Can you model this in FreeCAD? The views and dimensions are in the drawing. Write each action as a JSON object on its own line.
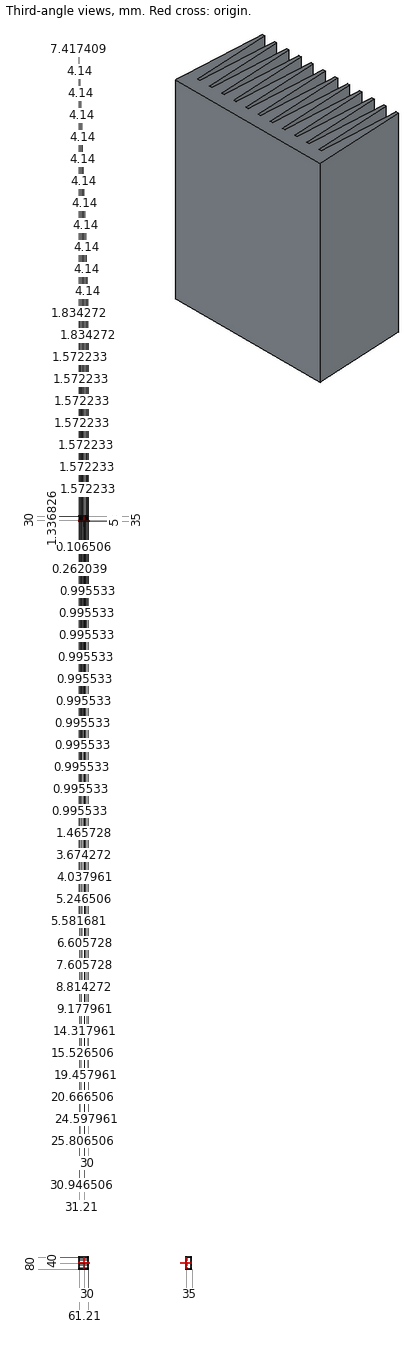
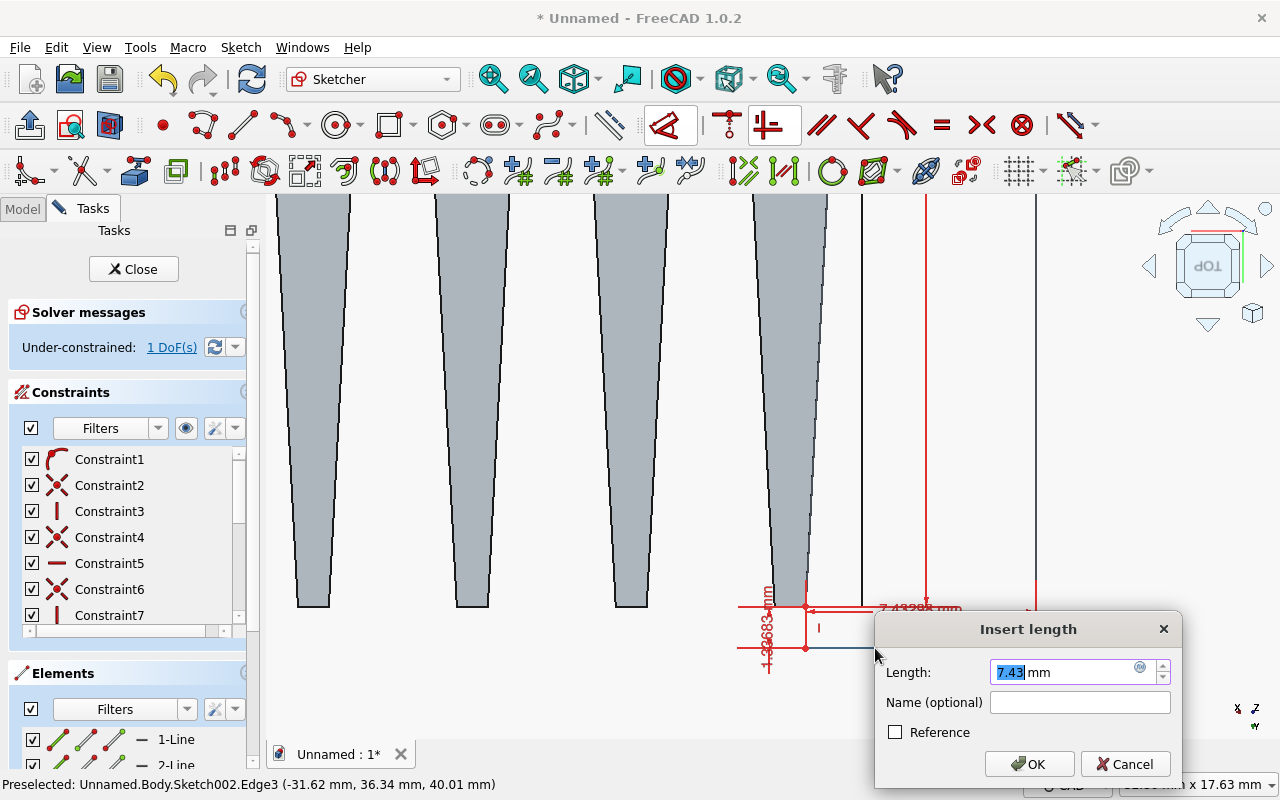
{"action": "type", "text": "7.417409"}
{"action": "key", "text": "Return"}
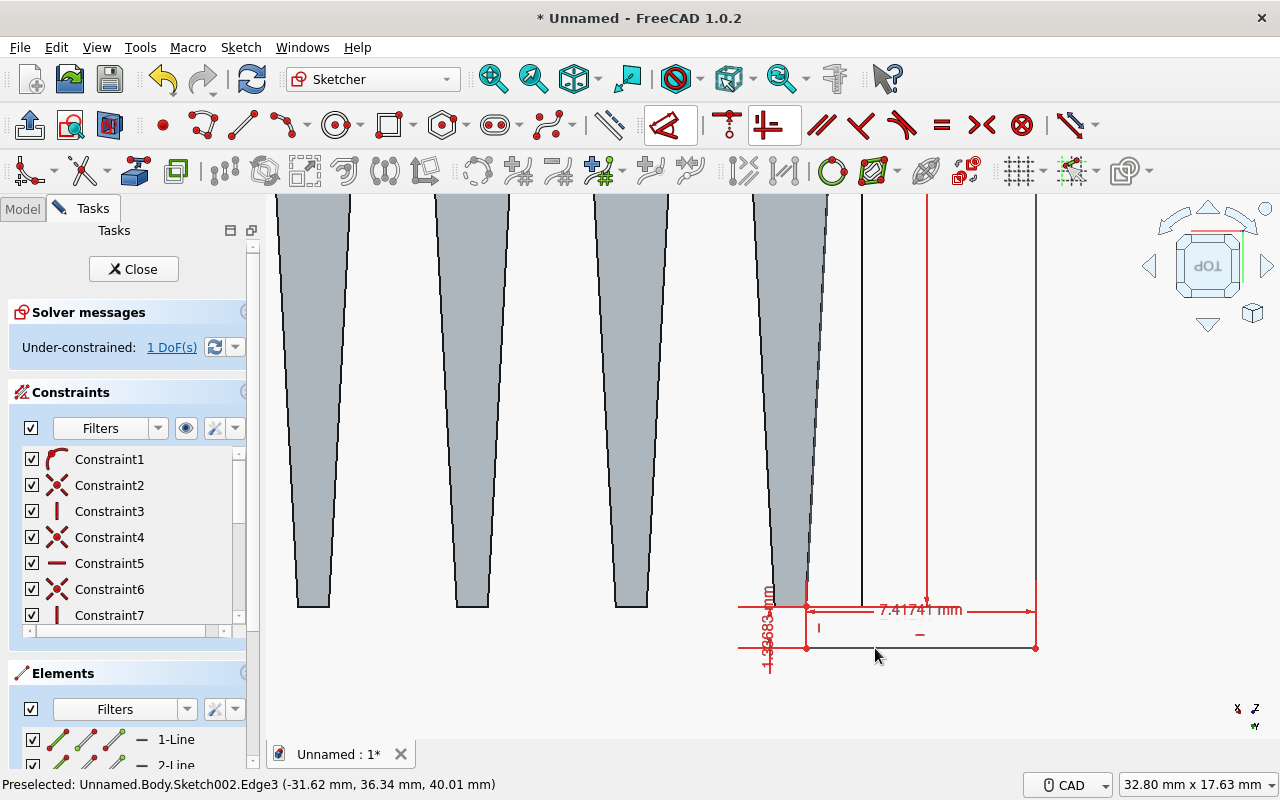
{"action": "scroll", "coordinate": [807, 630], "scroll_direction": "down", "scroll_amount": 6}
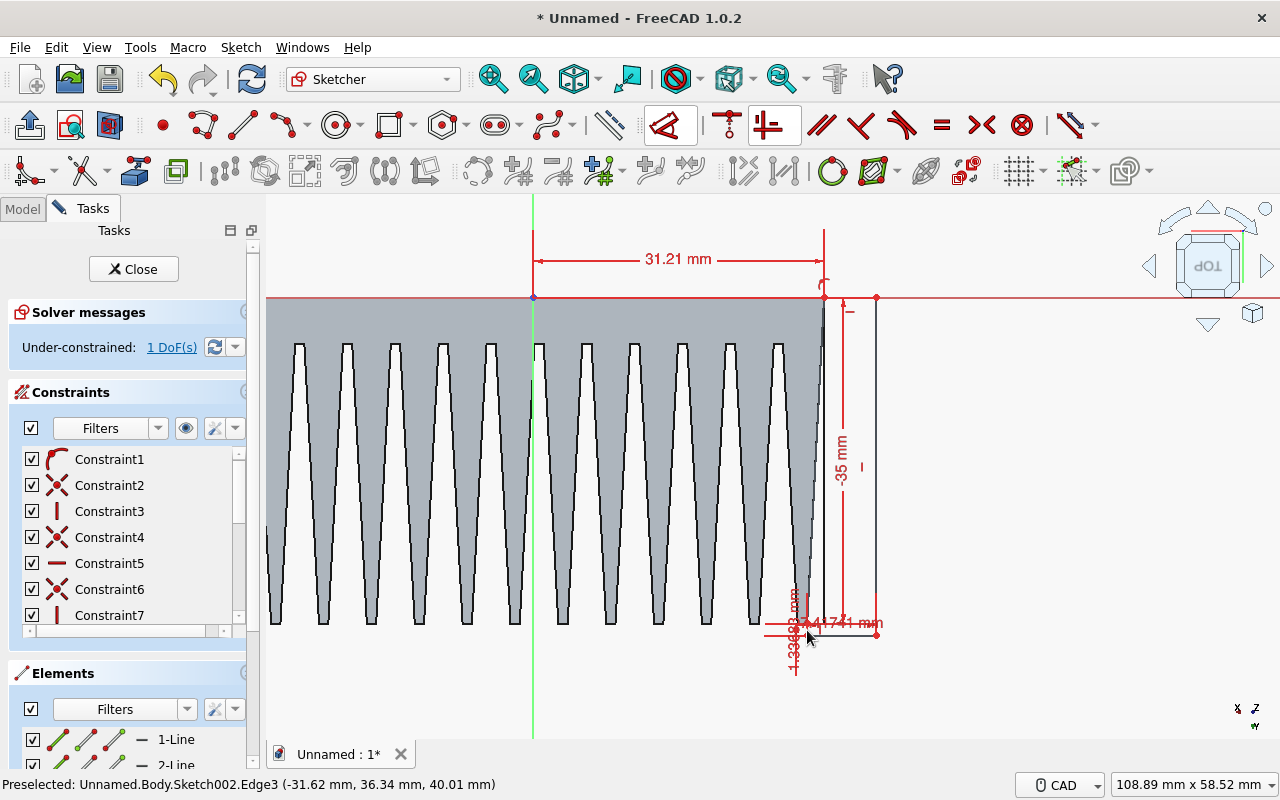
{"action": "left_click", "coordinate": [861, 298]}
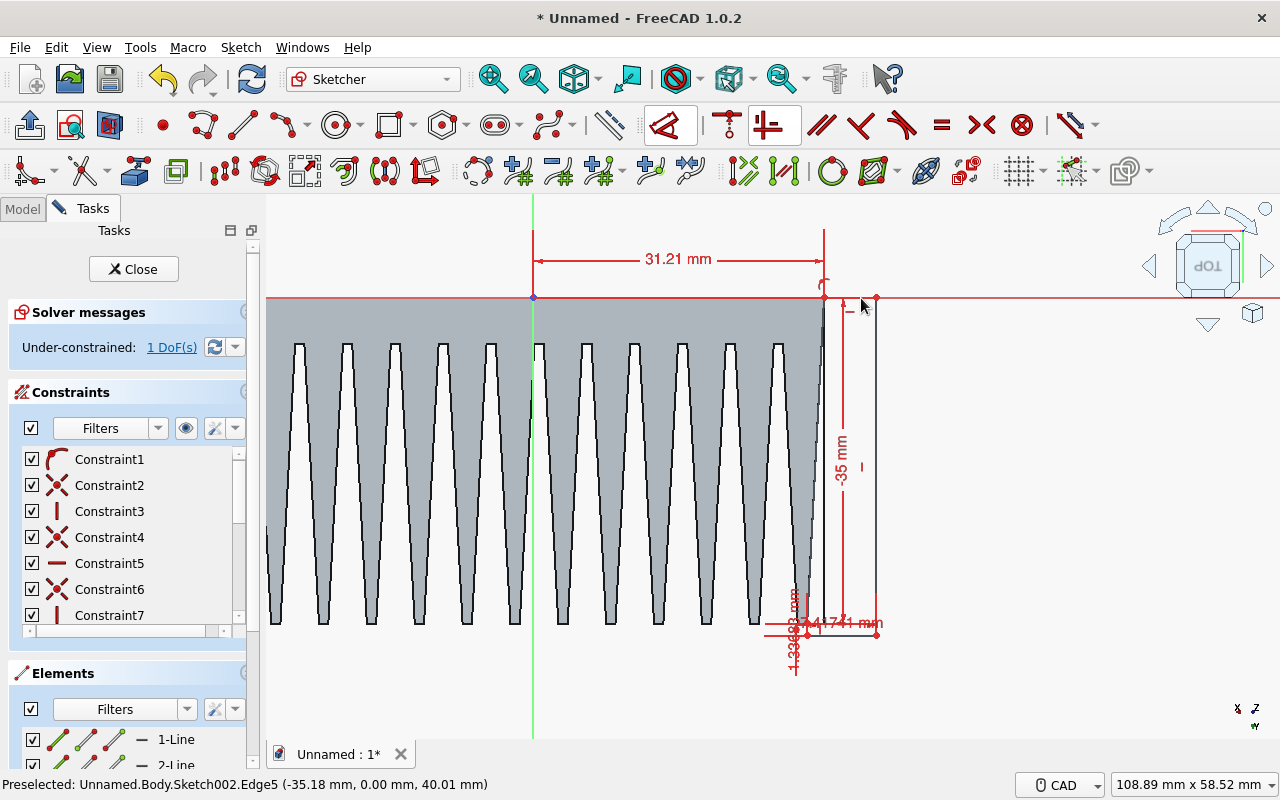
{"action": "key", "text": "l"}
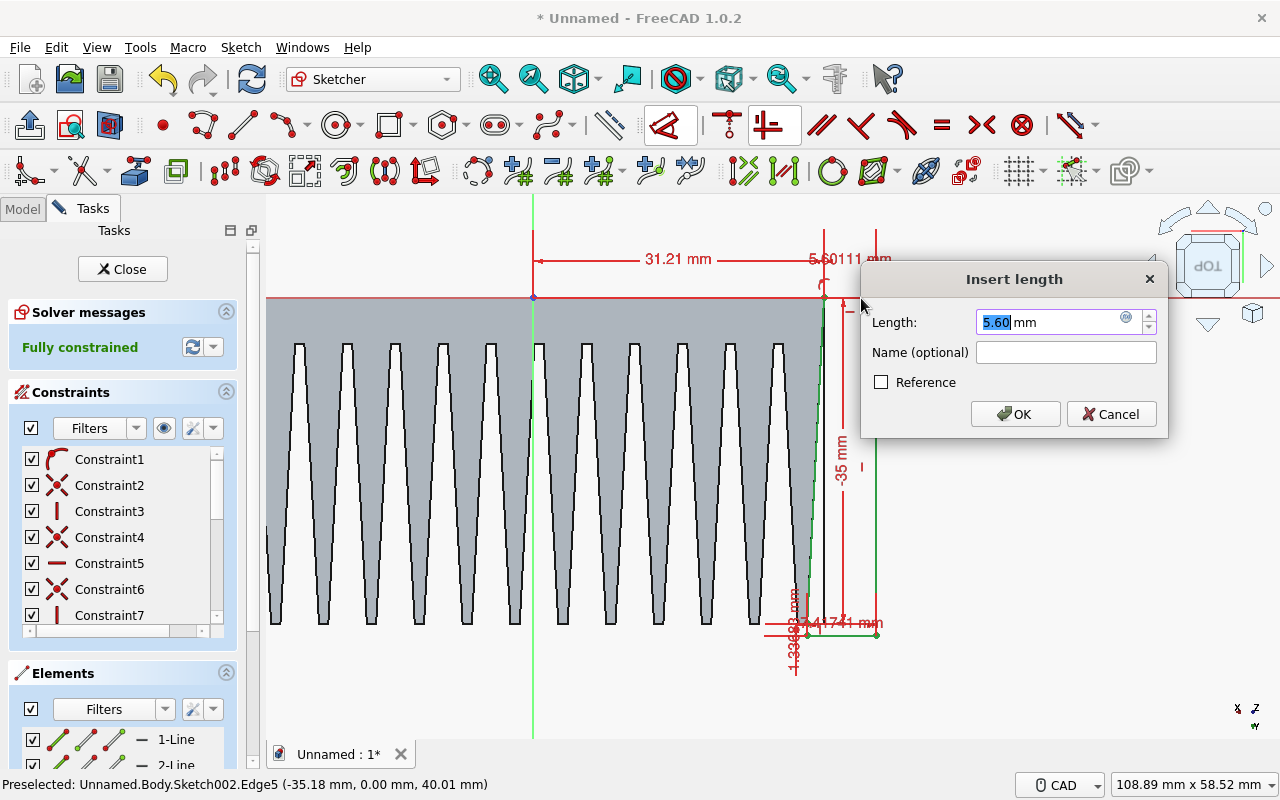
{"action": "type", "text": "5.581681"}
{"action": "key", "text": "Return"}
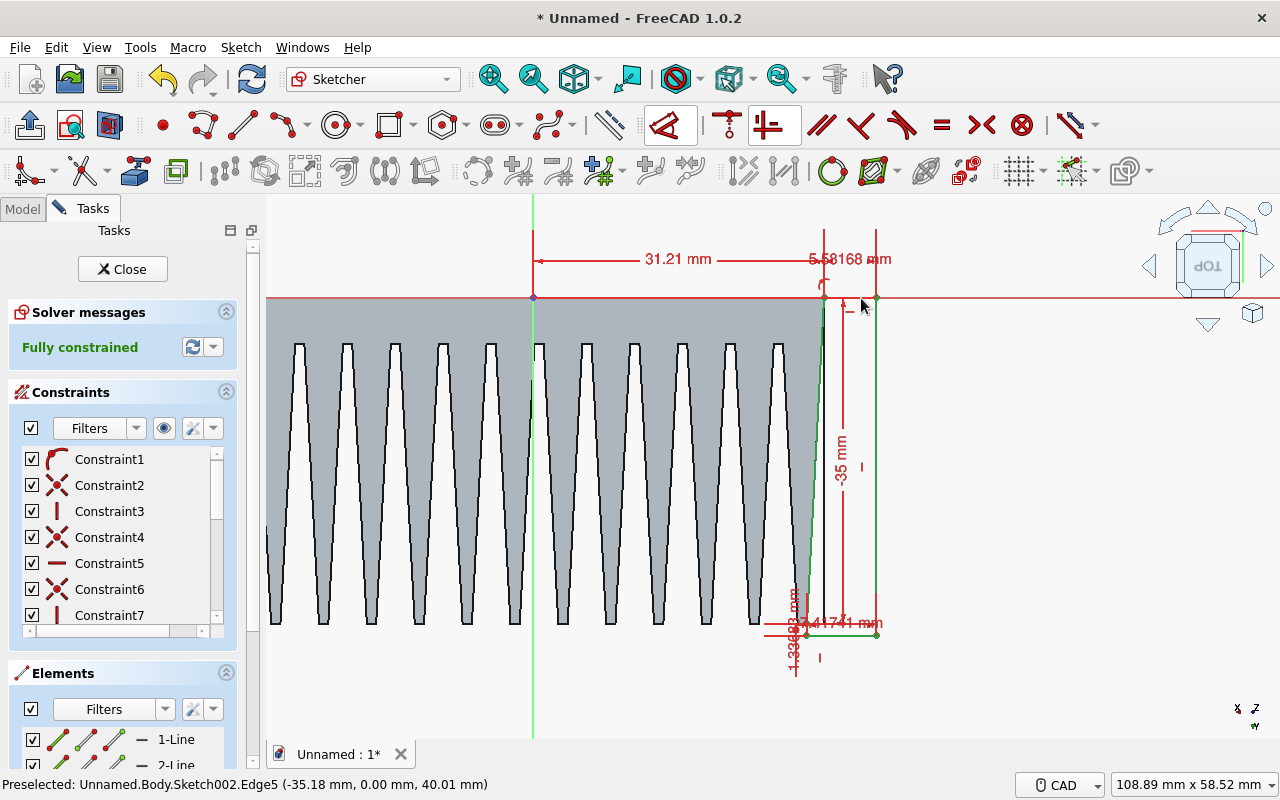
{"action": "left_click", "coordinate": [123, 269]}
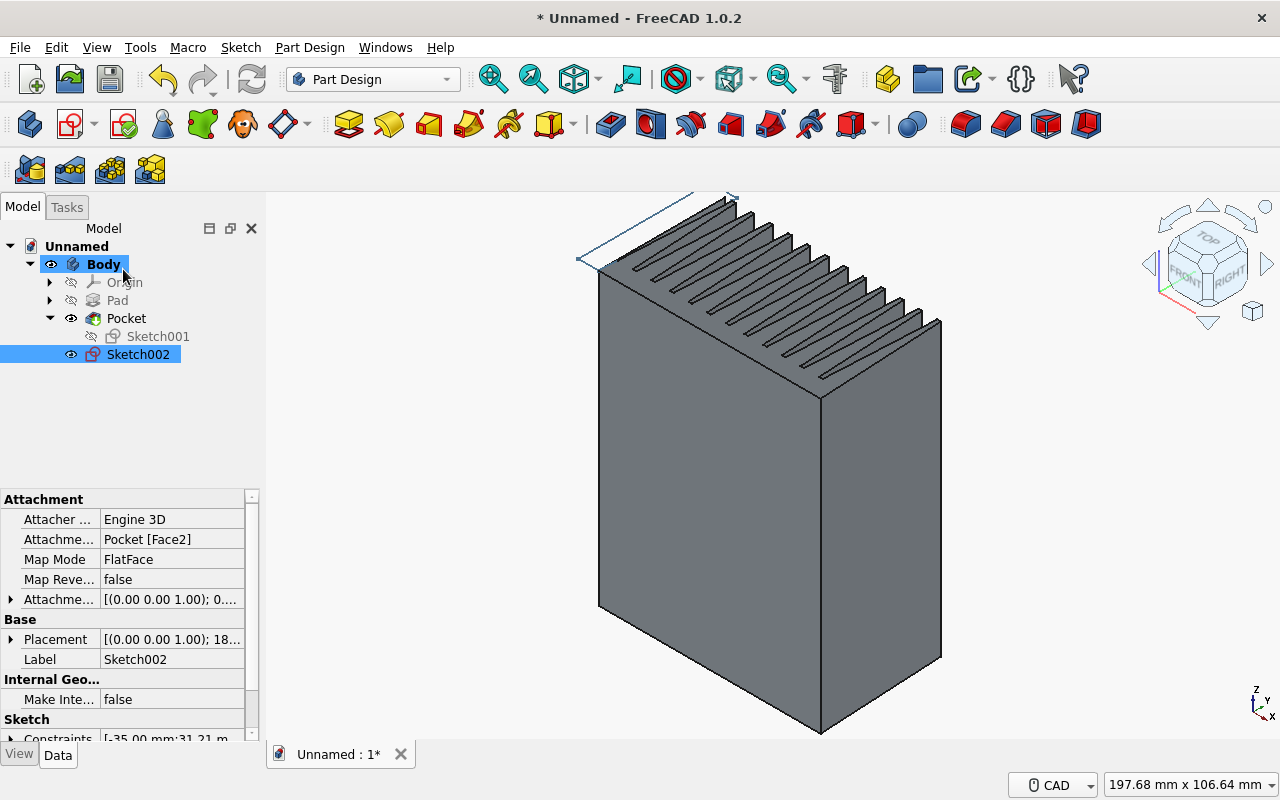
{"action": "left_click", "coordinate": [612, 124]}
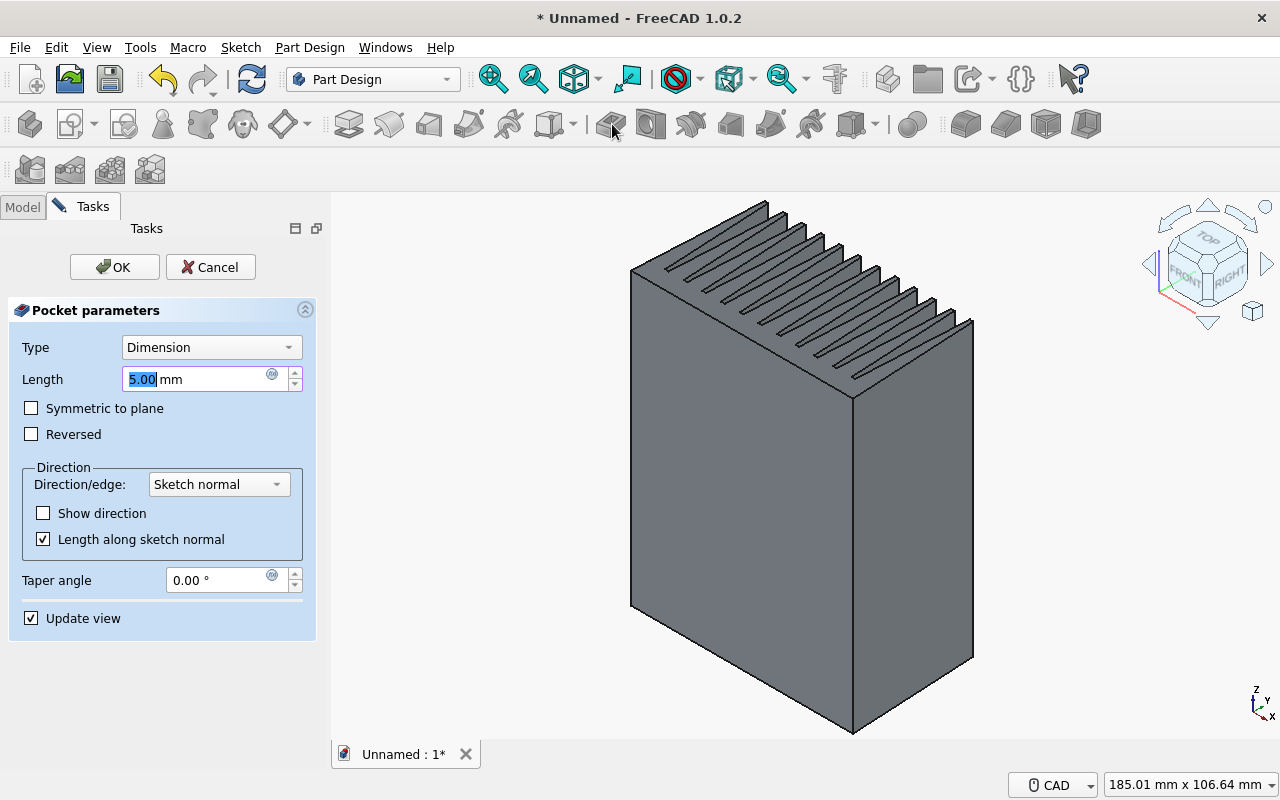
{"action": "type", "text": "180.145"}
{"action": "key", "text": "Tab"}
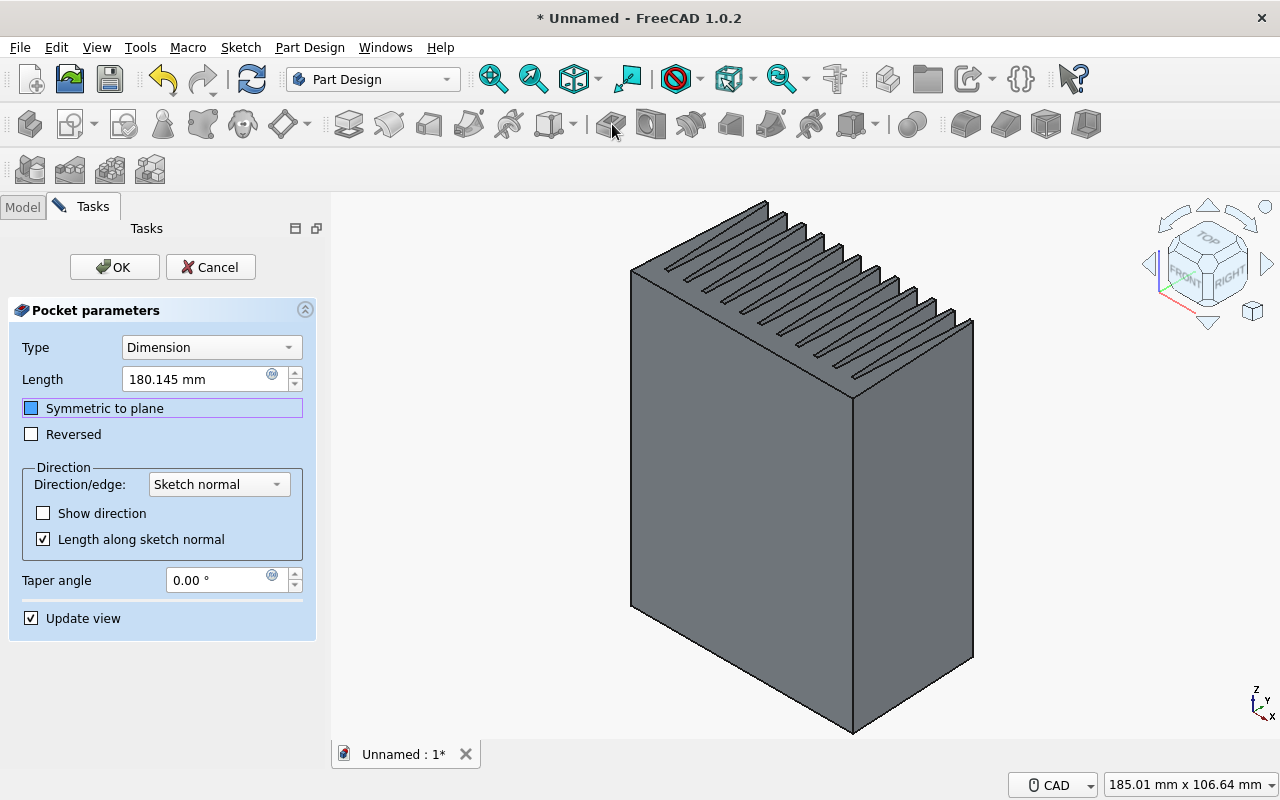
{"action": "left_click", "coordinate": [115, 267]}